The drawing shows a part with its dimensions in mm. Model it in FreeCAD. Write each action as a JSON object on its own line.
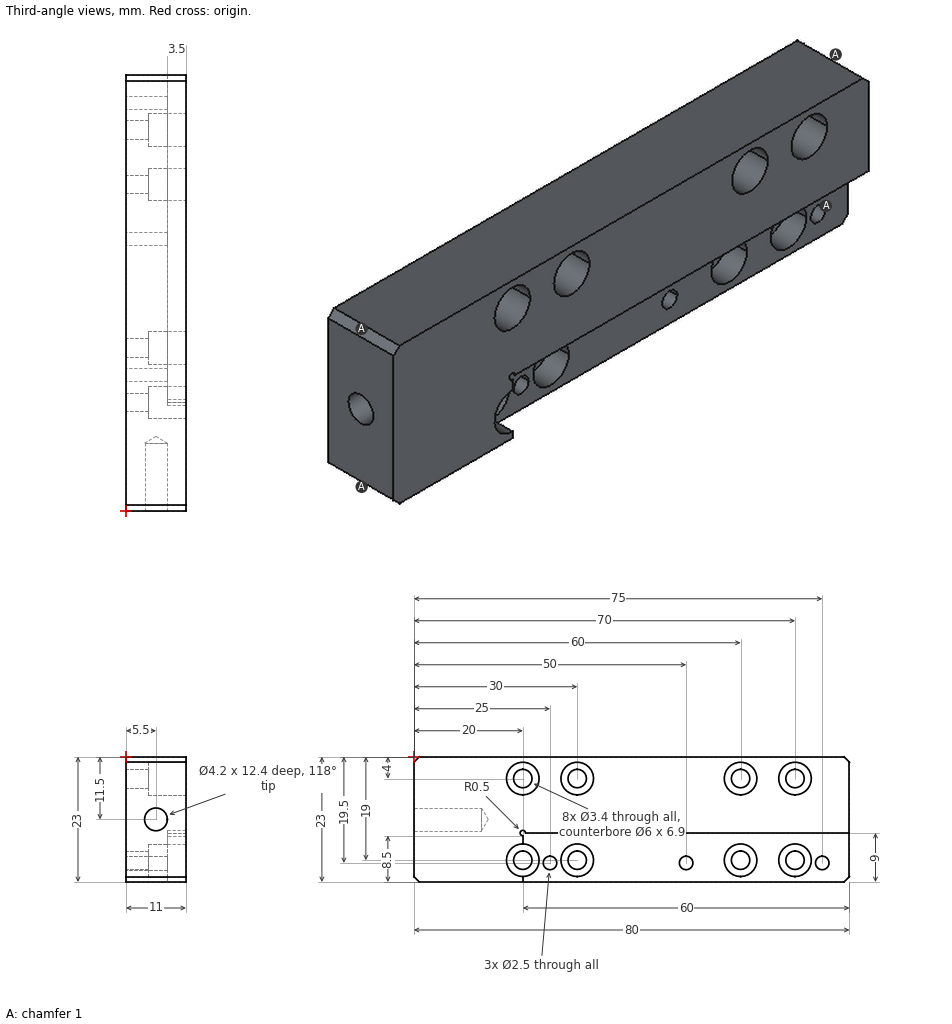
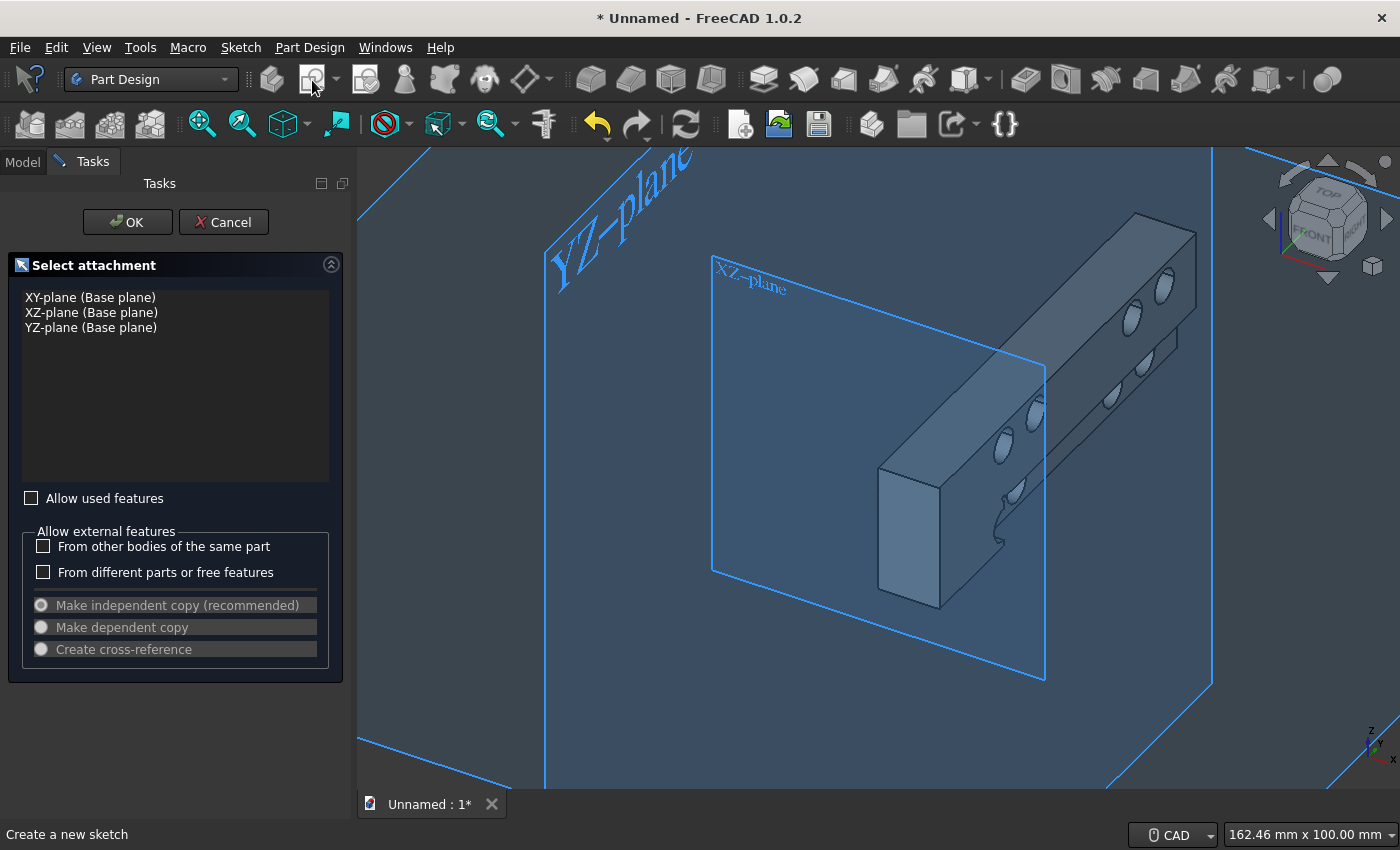
{"action": "left_click", "coordinate": [82, 312]}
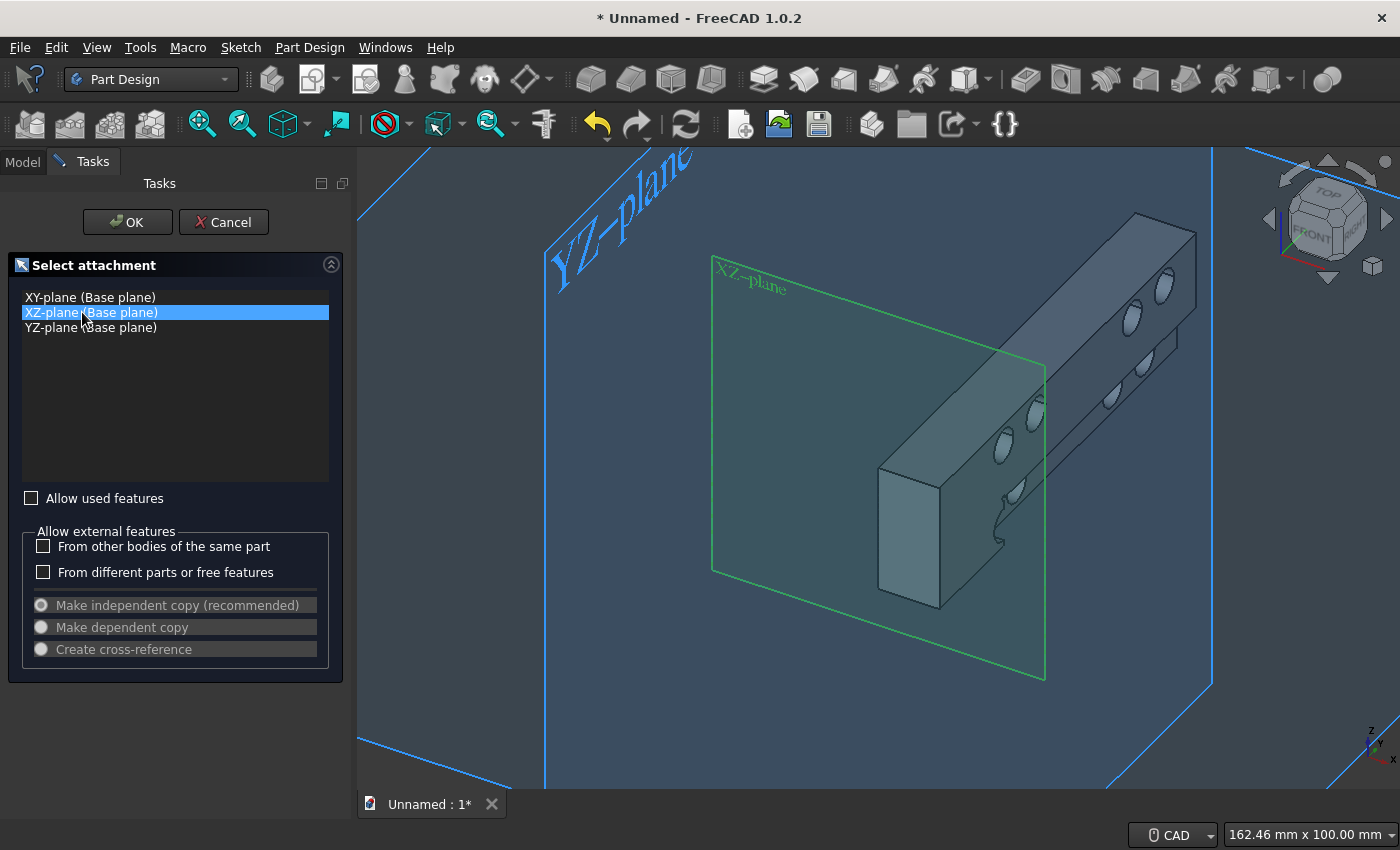
{"action": "left_click", "coordinate": [128, 222]}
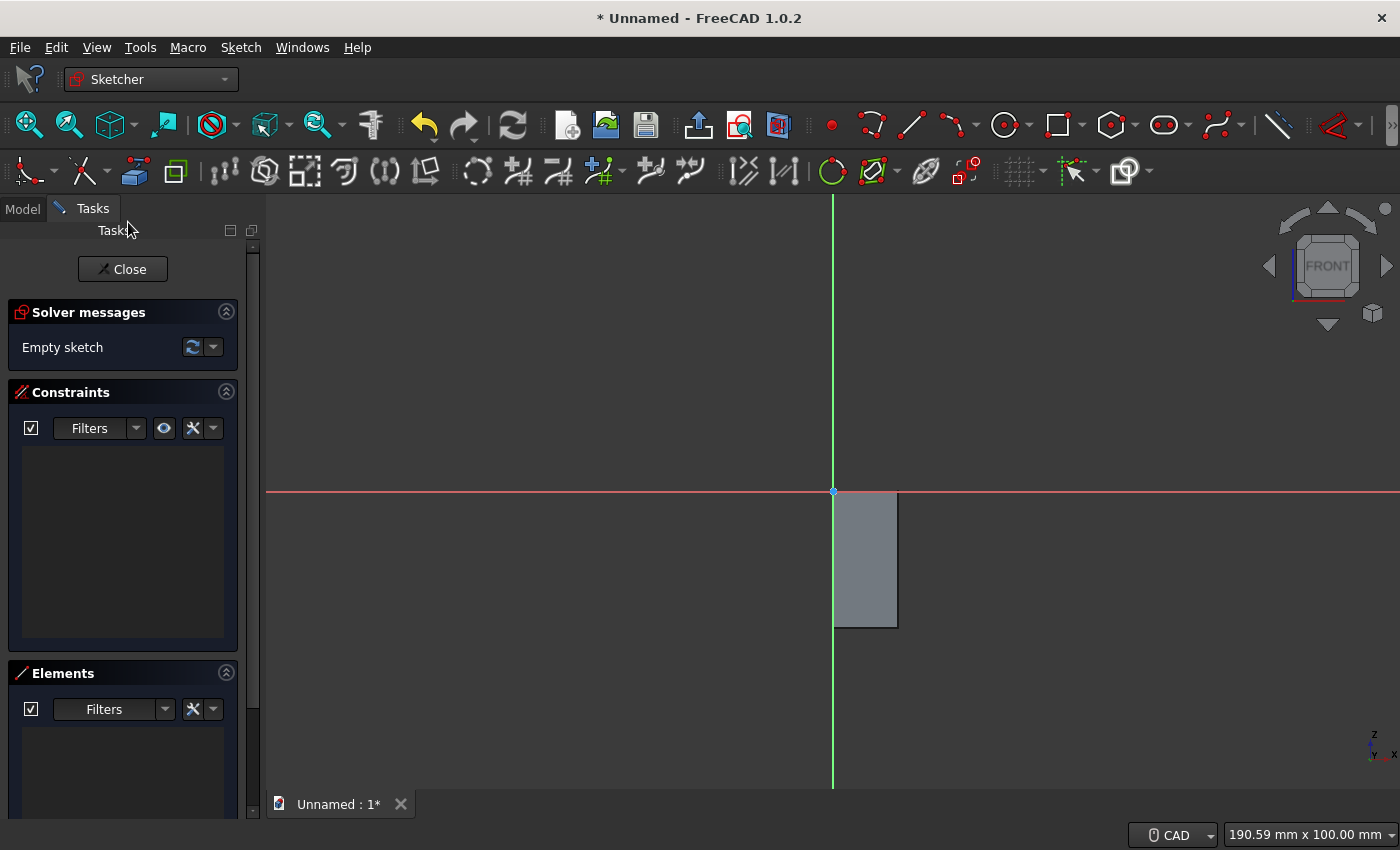
{"action": "scroll", "coordinate": [872, 564], "scroll_direction": "up", "scroll_amount": 14}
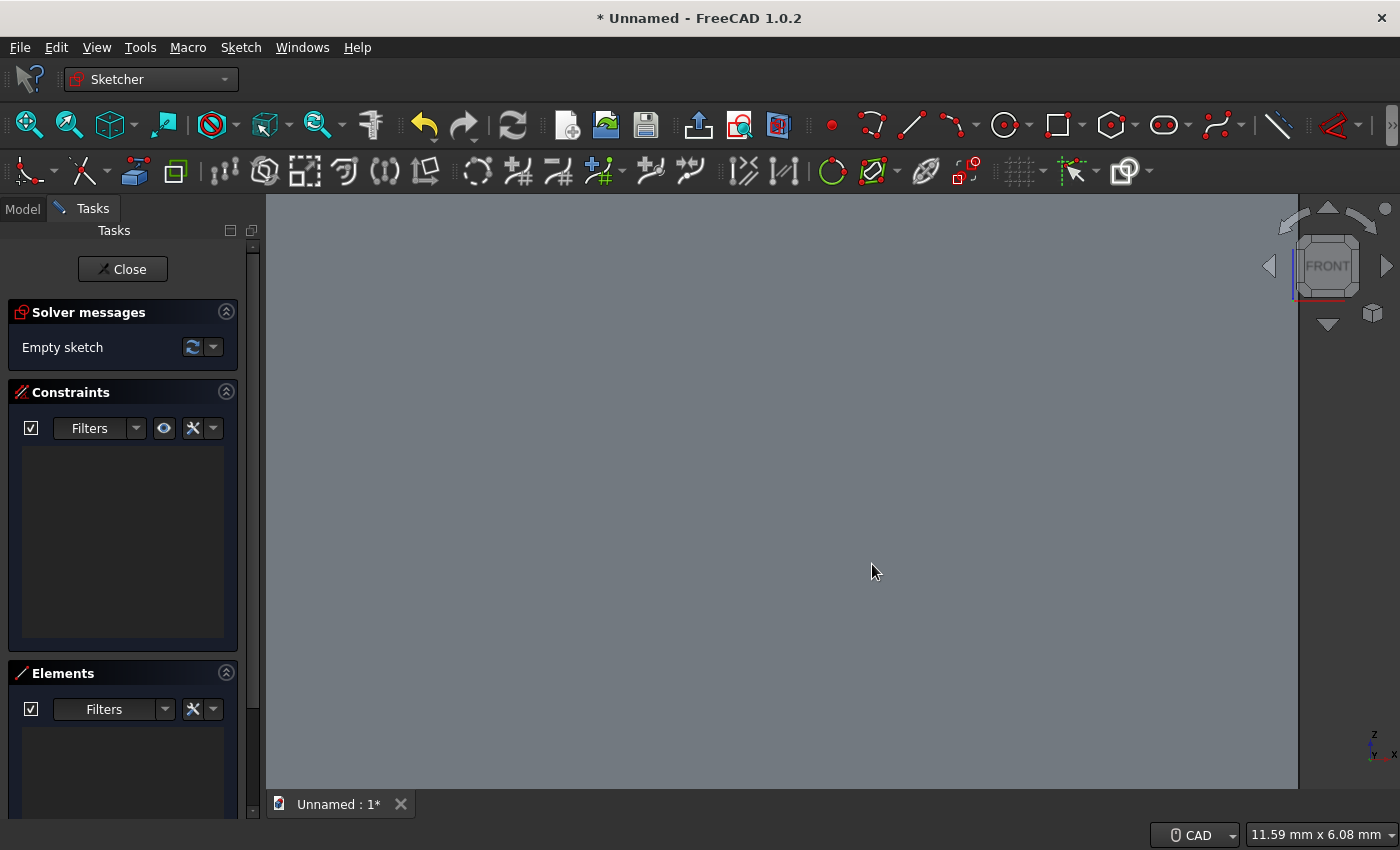
{"action": "left_click", "coordinate": [1006, 126]}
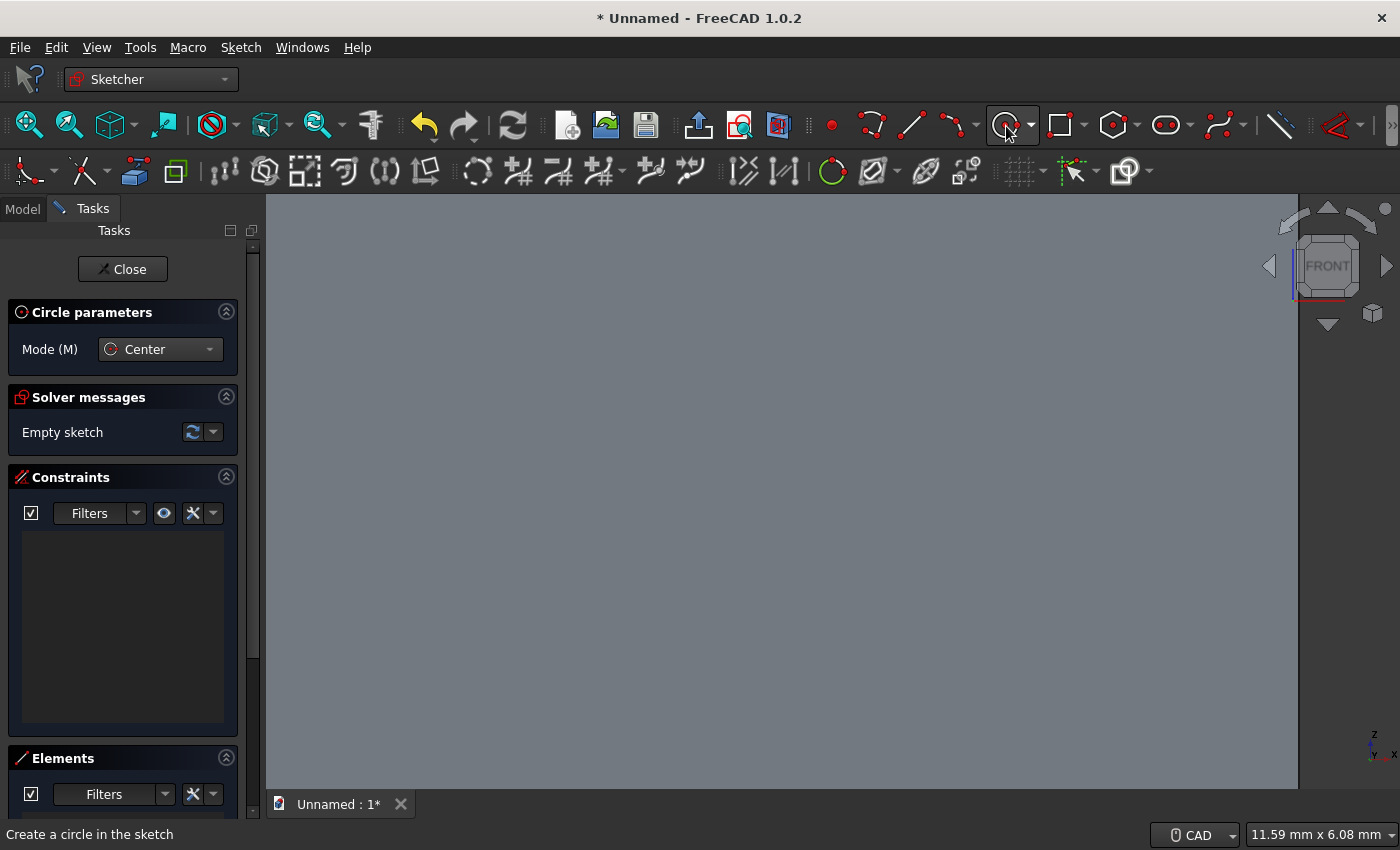
{"action": "left_click", "coordinate": [761, 487]}
{"action": "left_click", "coordinate": [906, 342]}
{"action": "key", "text": "Escape"}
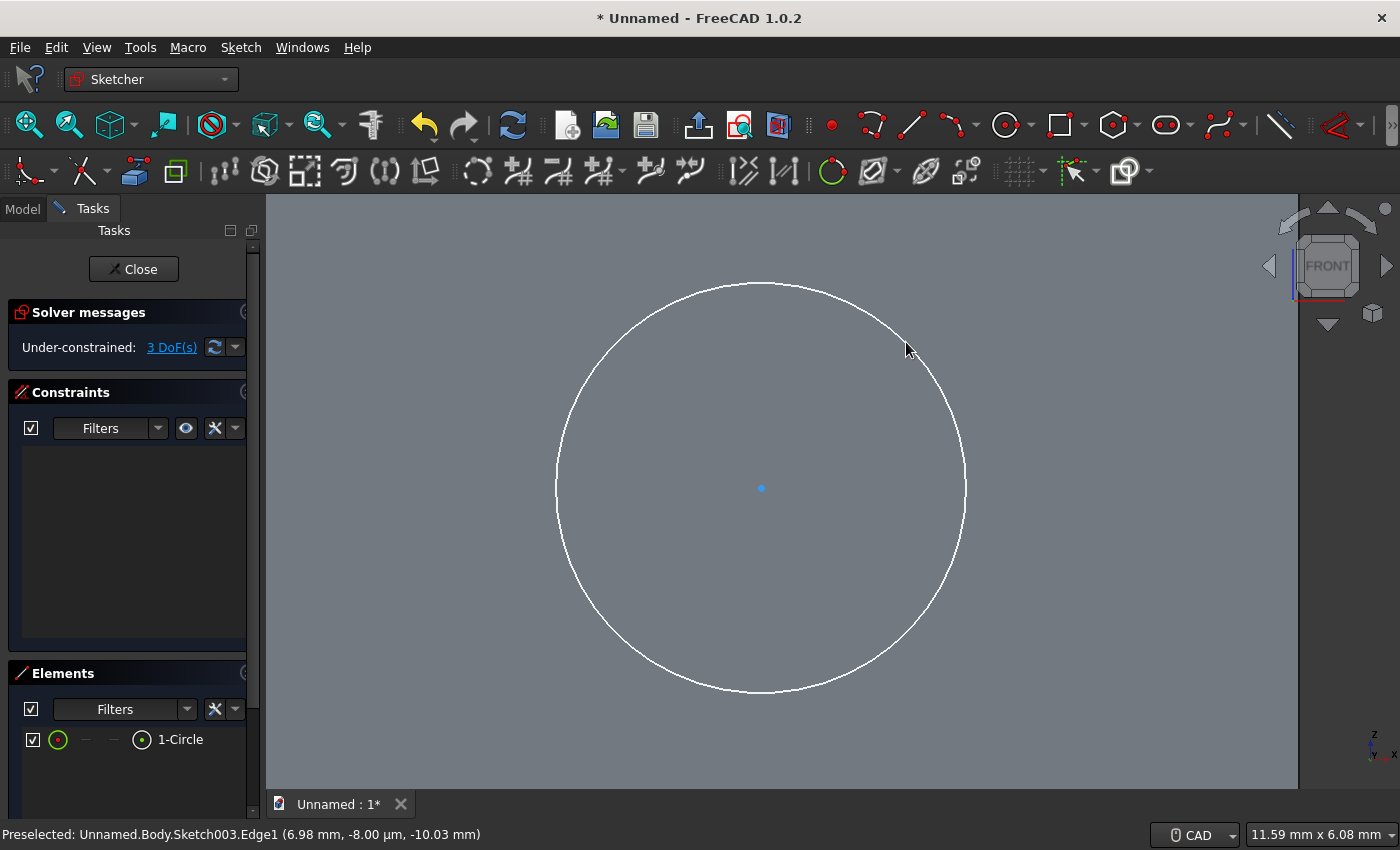
{"action": "left_click", "coordinate": [1336, 126]}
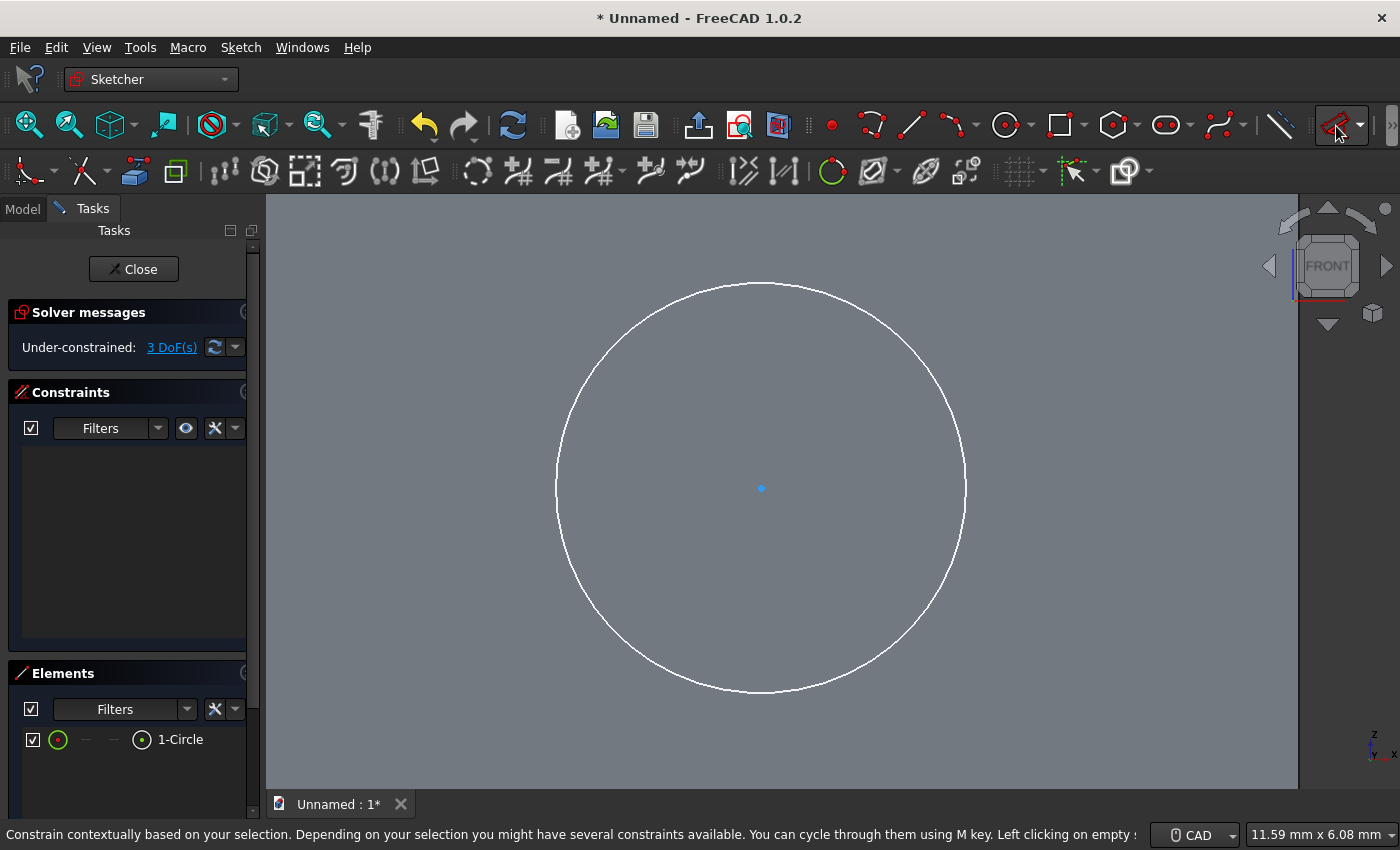
{"action": "left_click", "coordinate": [906, 343]}
{"action": "left_click", "coordinate": [929, 320]}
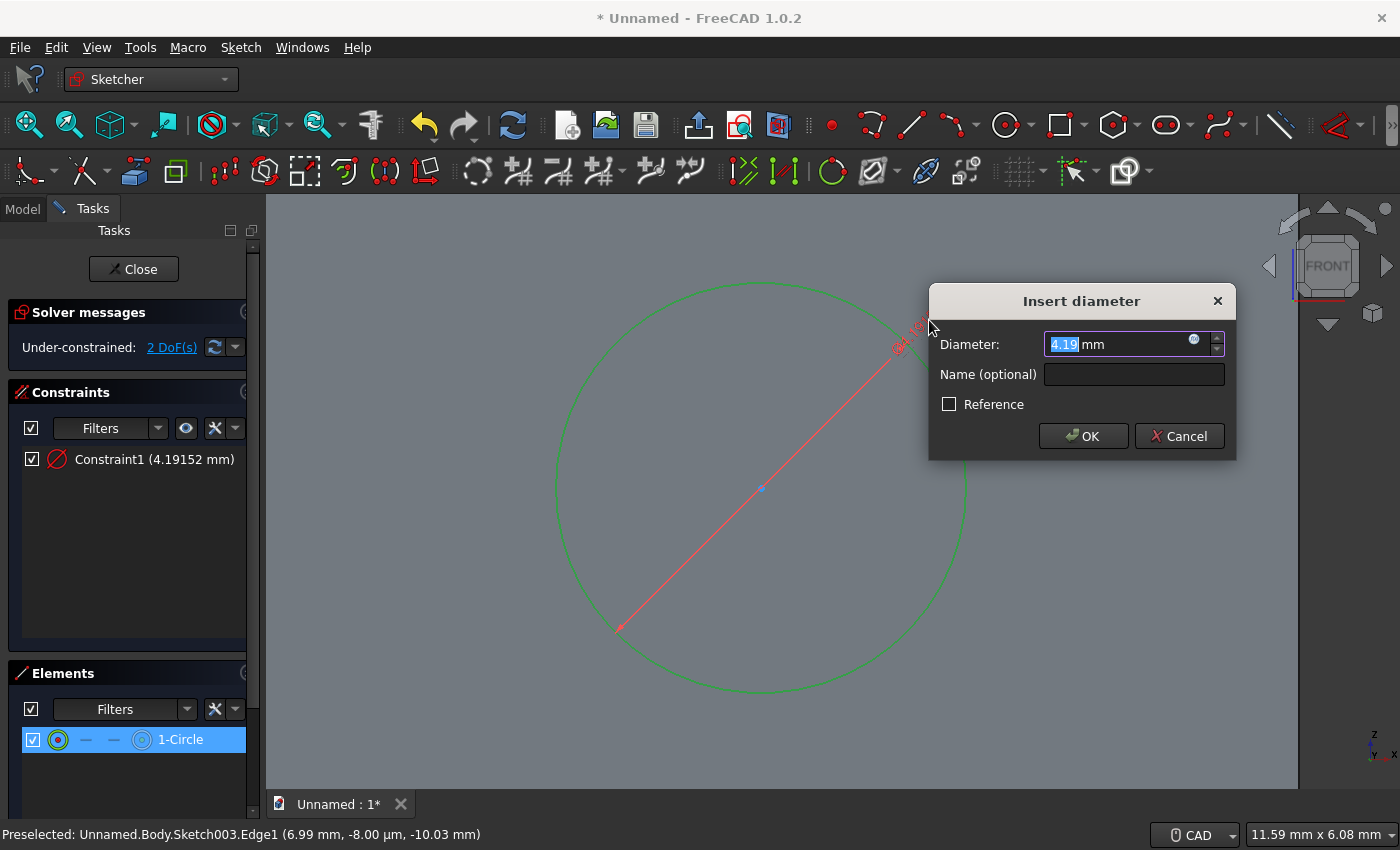
{"action": "type", "text": "4.2"}
{"action": "key", "text": "Return"}